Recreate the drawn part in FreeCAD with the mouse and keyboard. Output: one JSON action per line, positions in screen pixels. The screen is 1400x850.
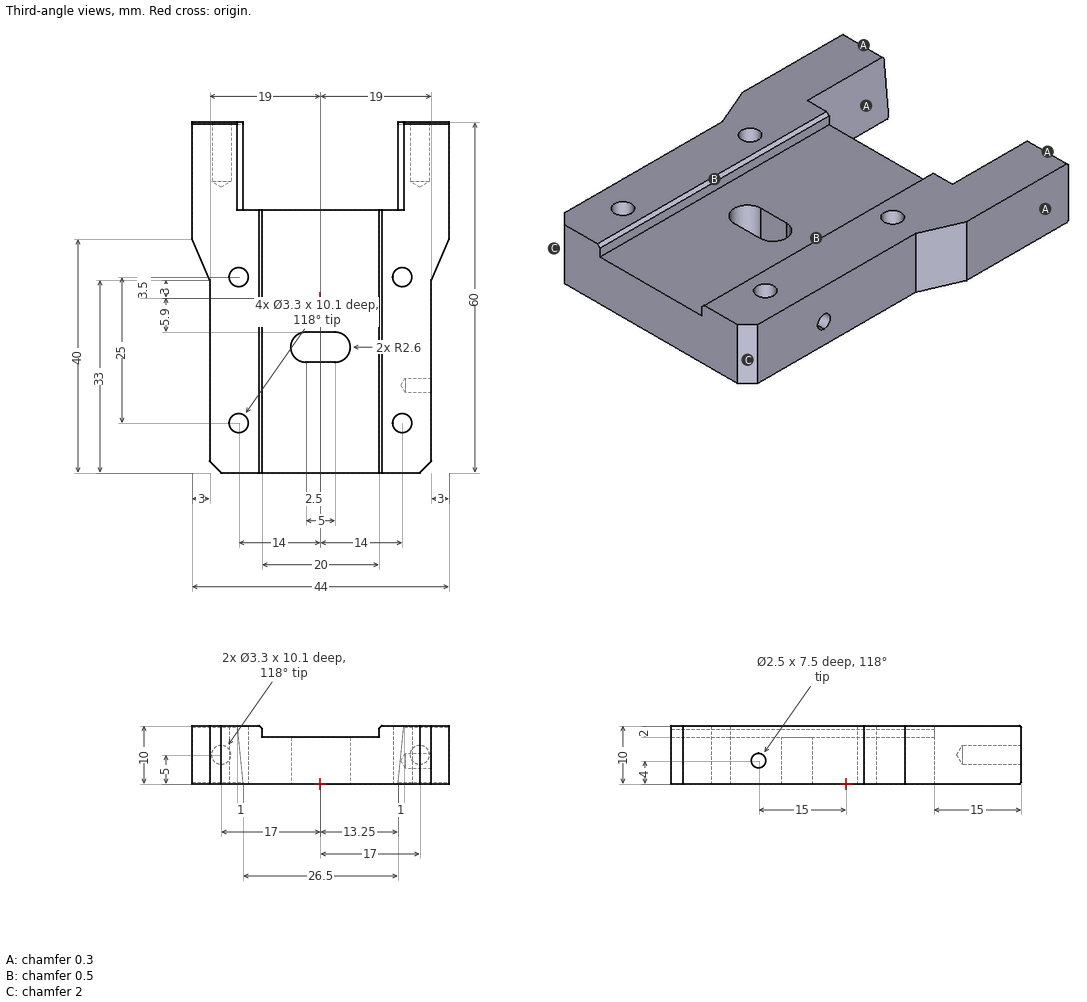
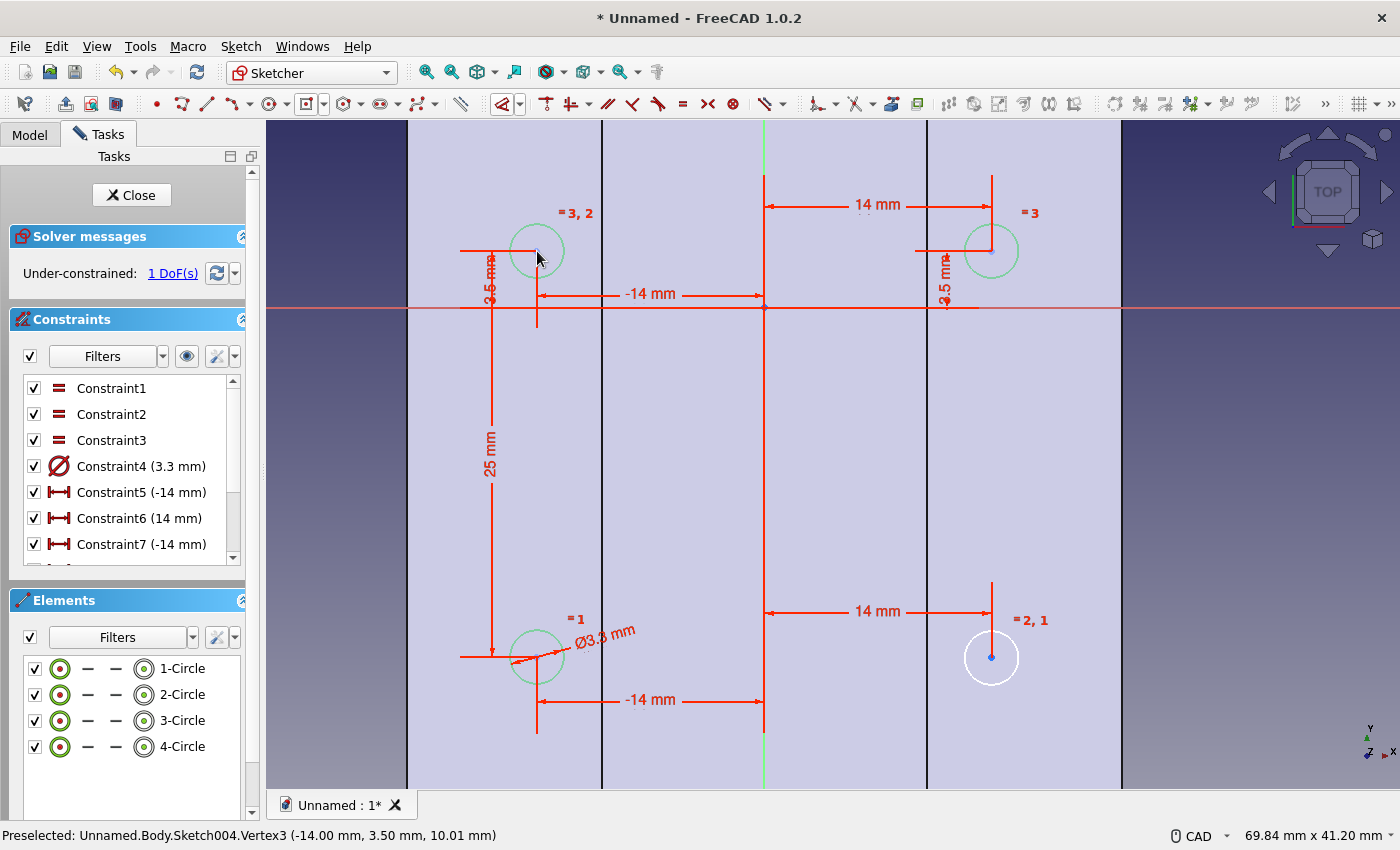
{"action": "left_click", "coordinate": [992, 658]}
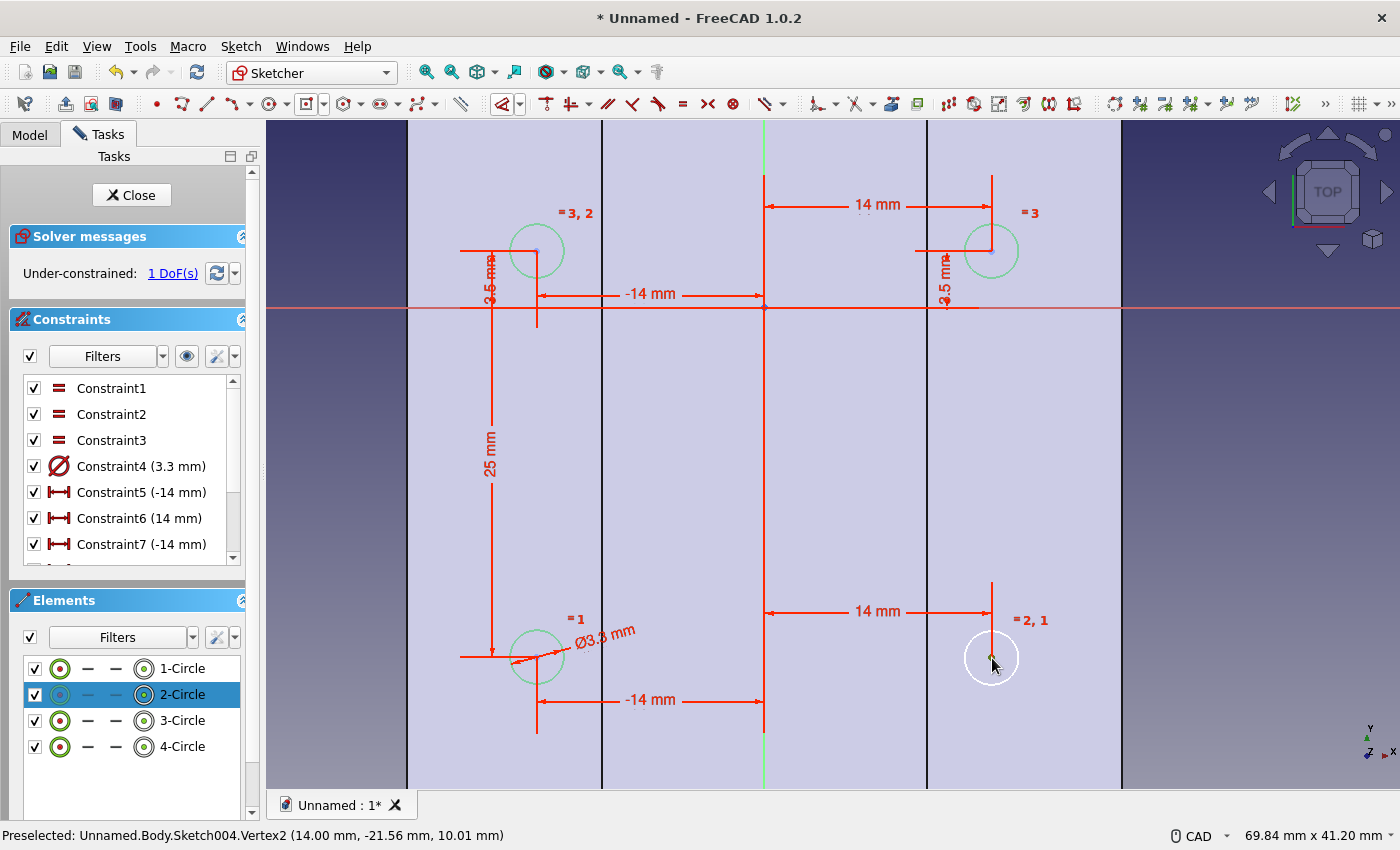
{"action": "left_click", "coordinate": [537, 251]}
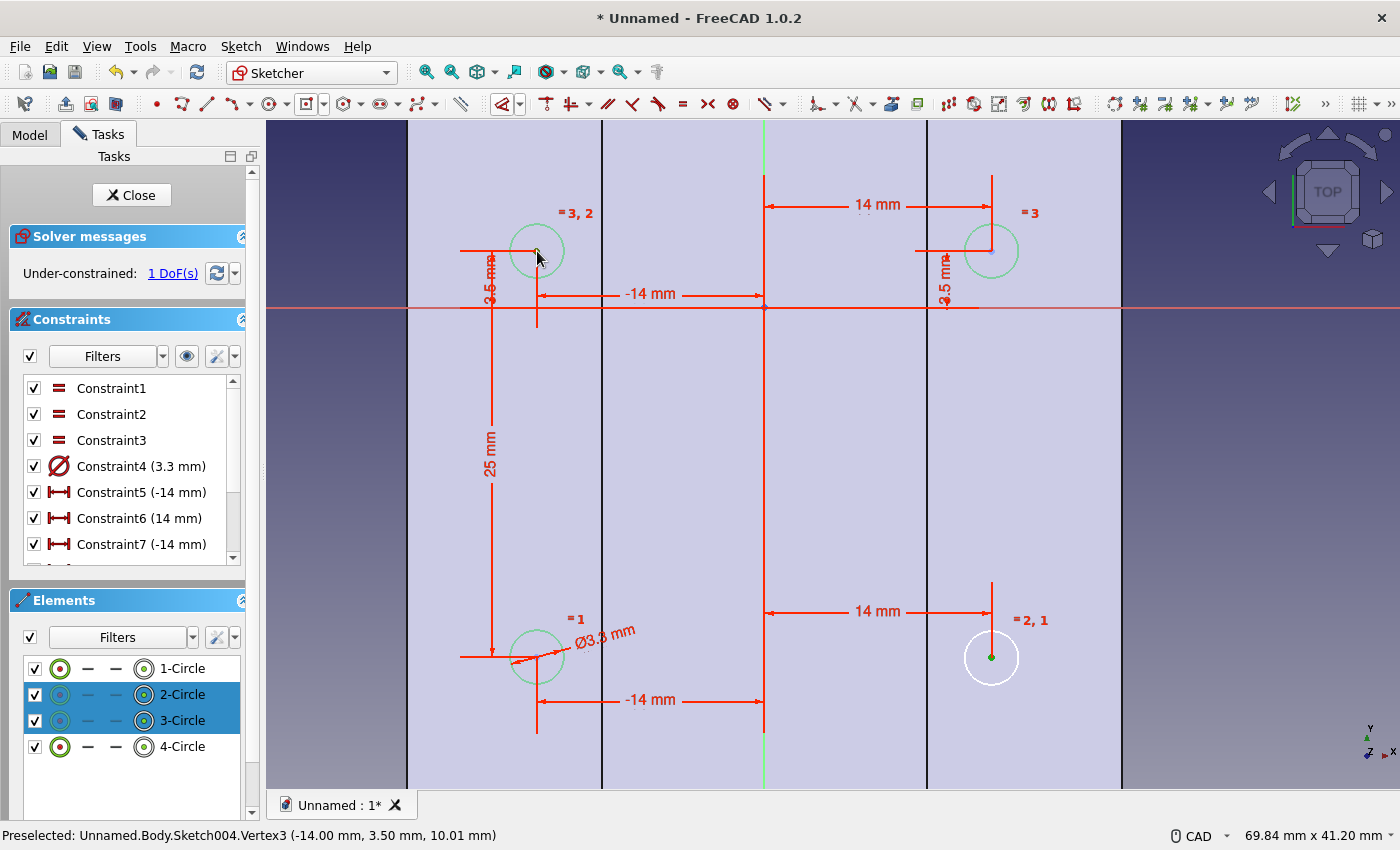
{"action": "key", "text": "i"}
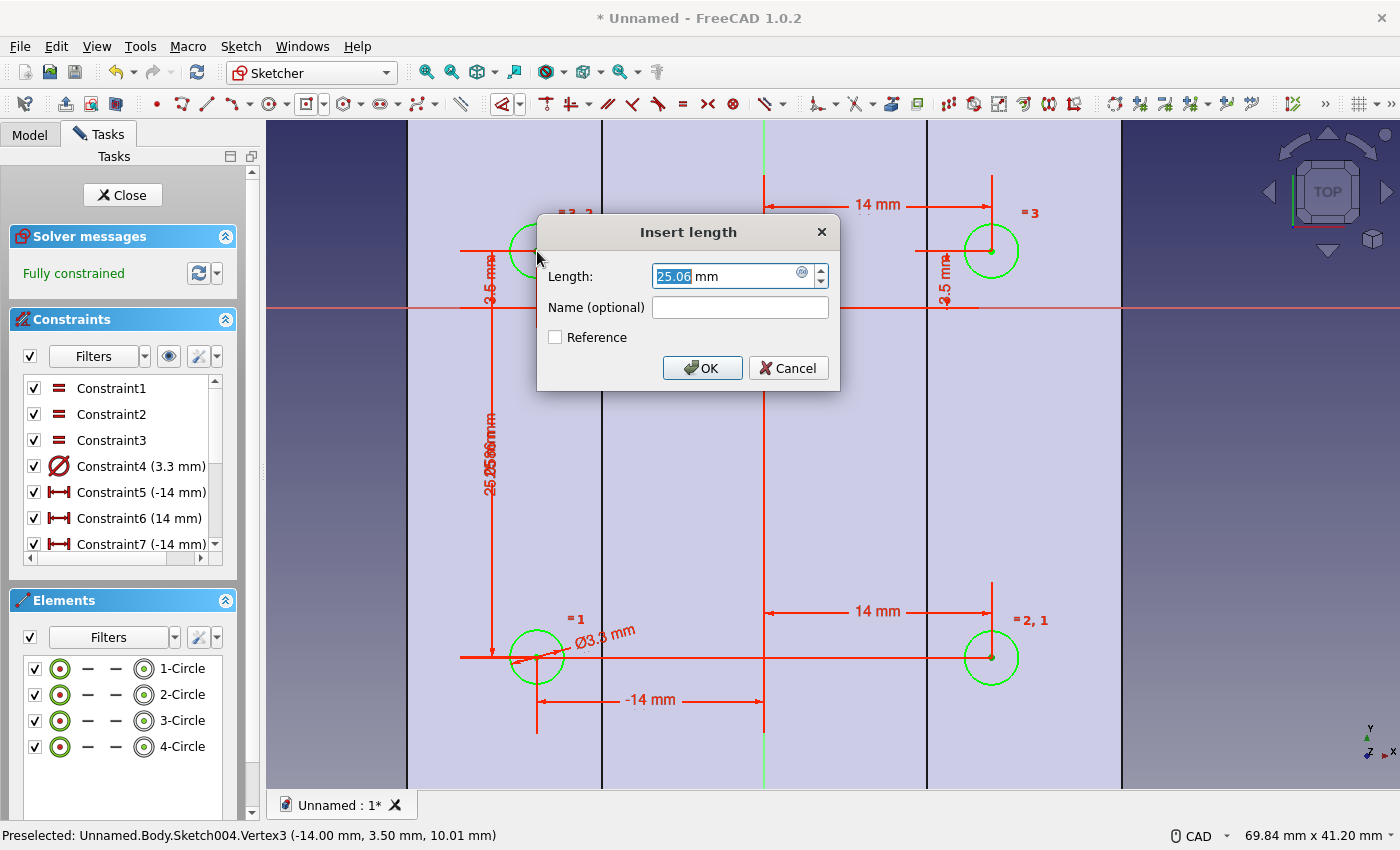
{"action": "type", "text": "25"}
{"action": "key", "text": "Return"}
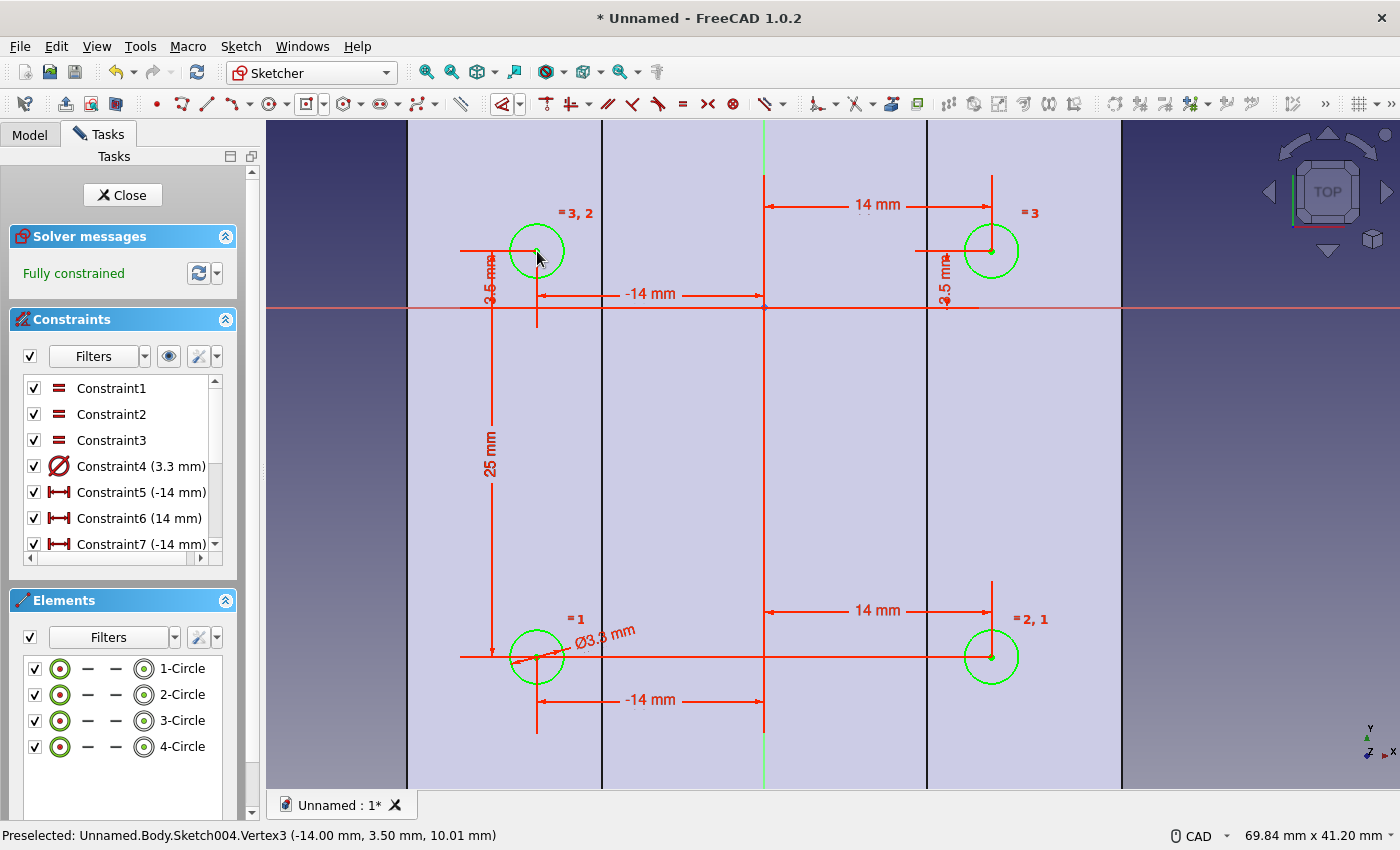
{"action": "left_click", "coordinate": [123, 195]}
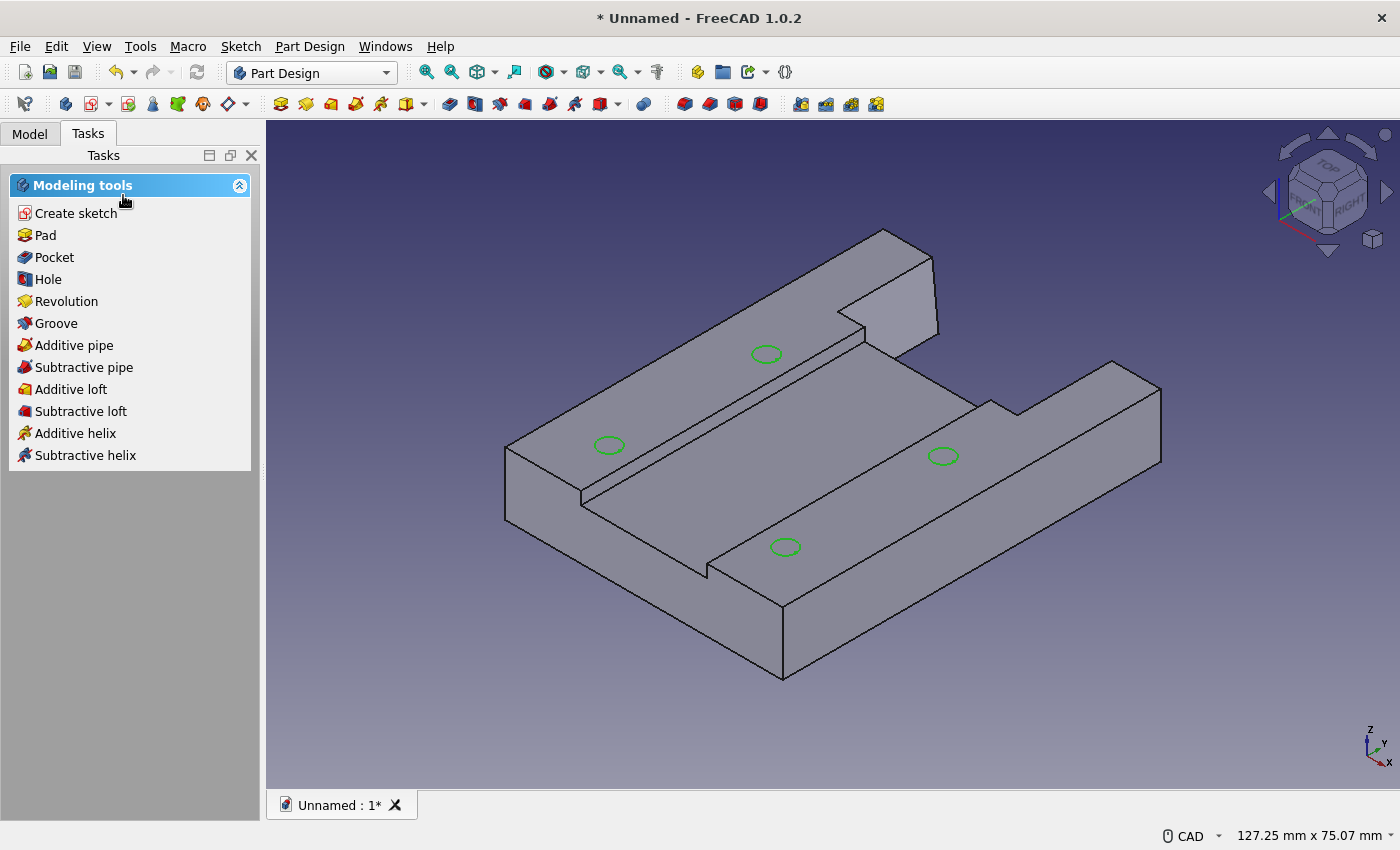
{"action": "left_click", "coordinate": [475, 104]}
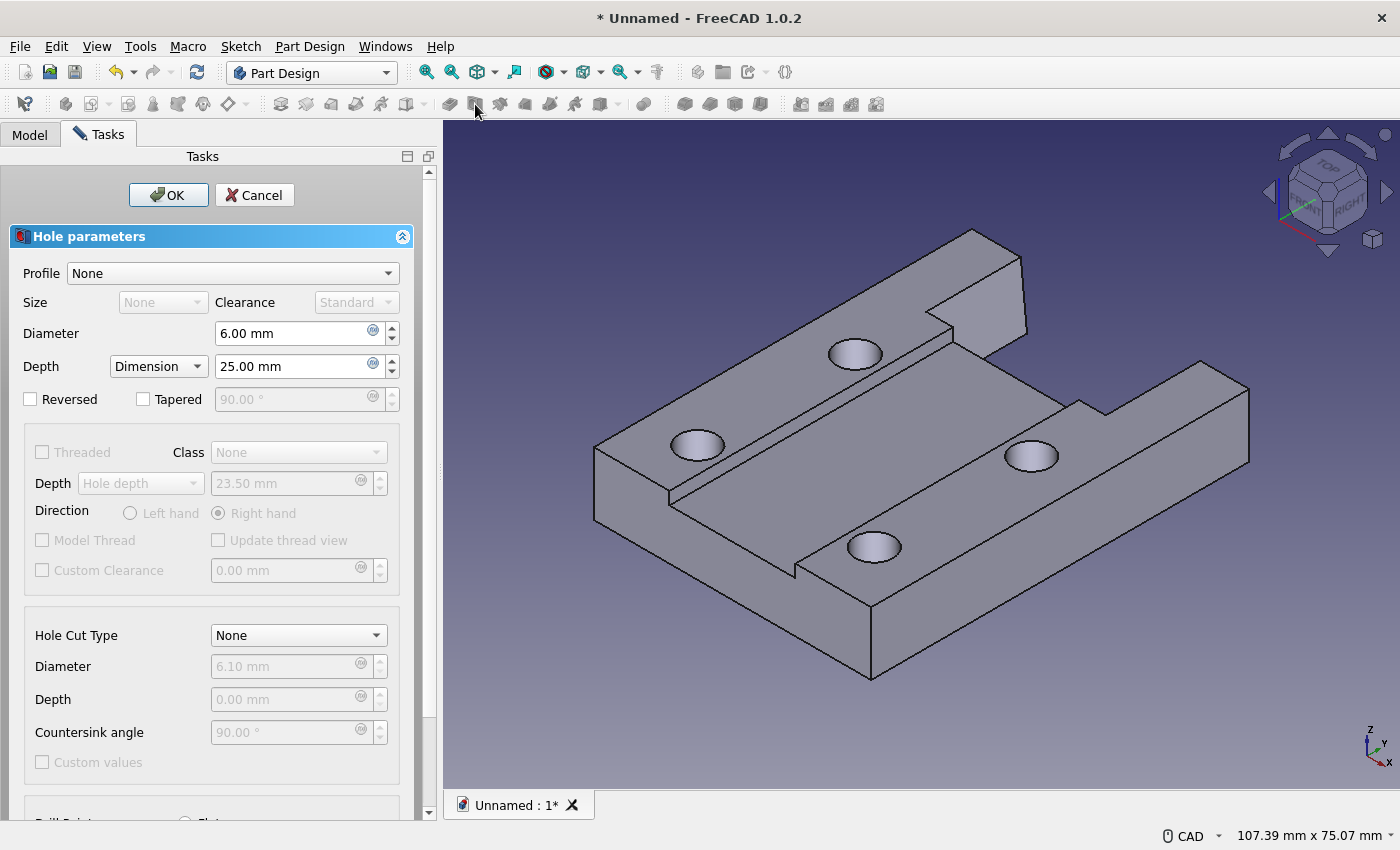
{"action": "triple_click", "coordinate": [300, 334]}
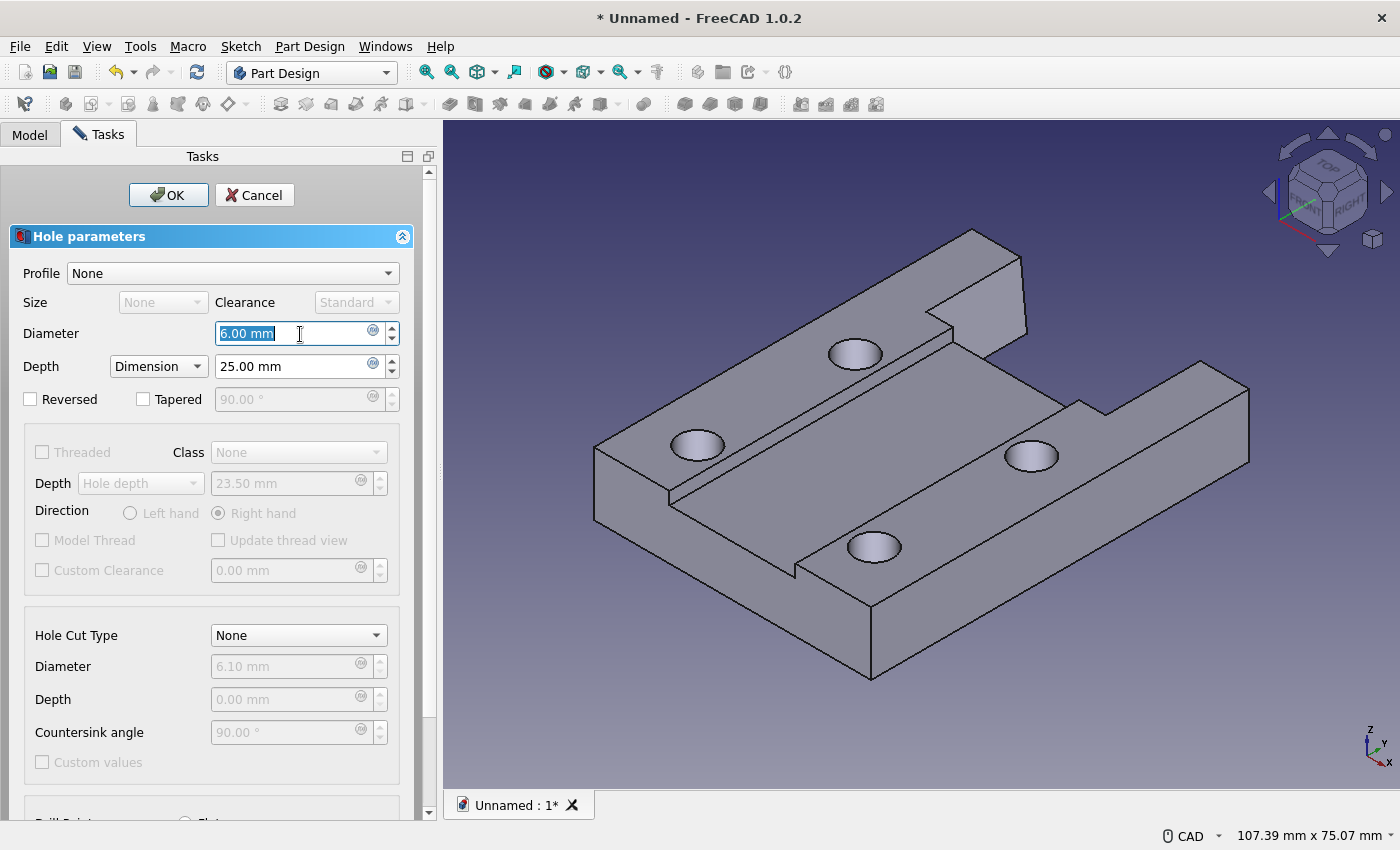
{"action": "type", "text": "3.3"}
{"action": "key", "text": "Tab"}